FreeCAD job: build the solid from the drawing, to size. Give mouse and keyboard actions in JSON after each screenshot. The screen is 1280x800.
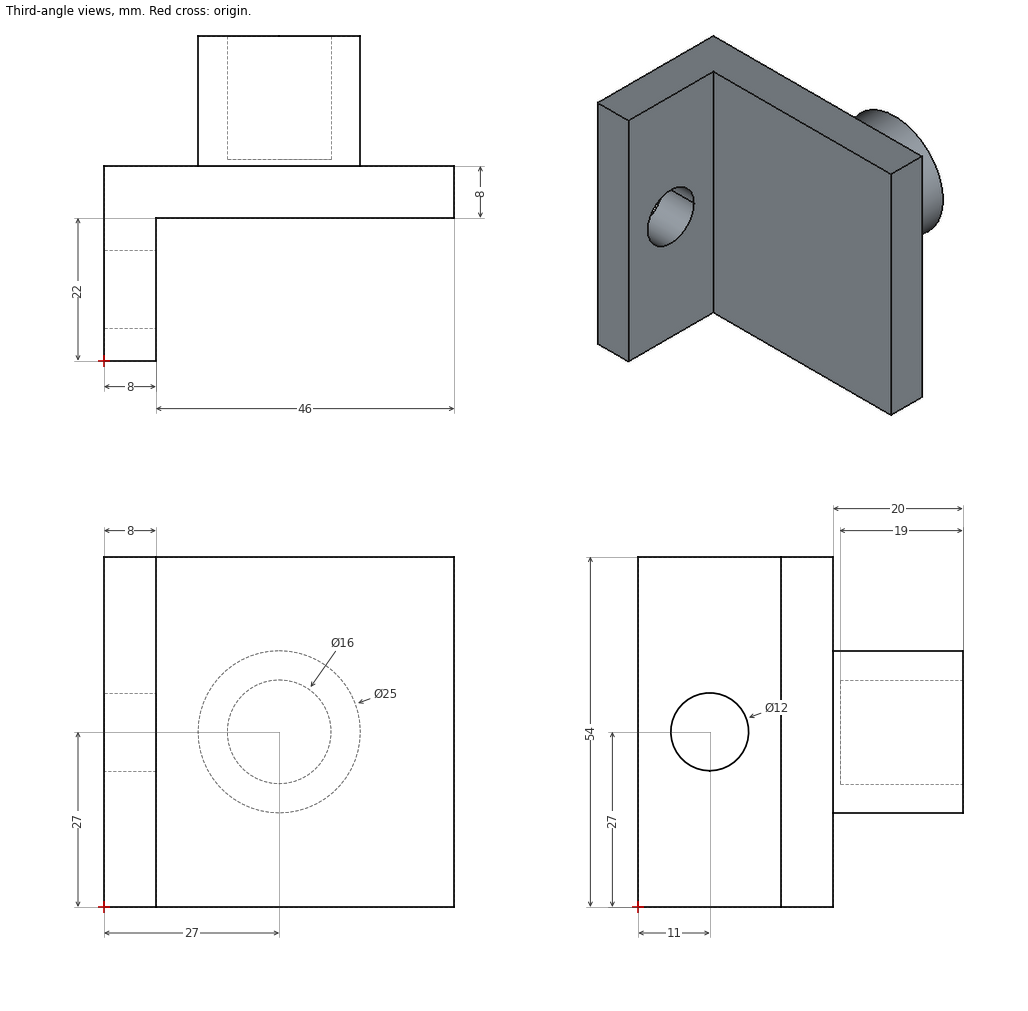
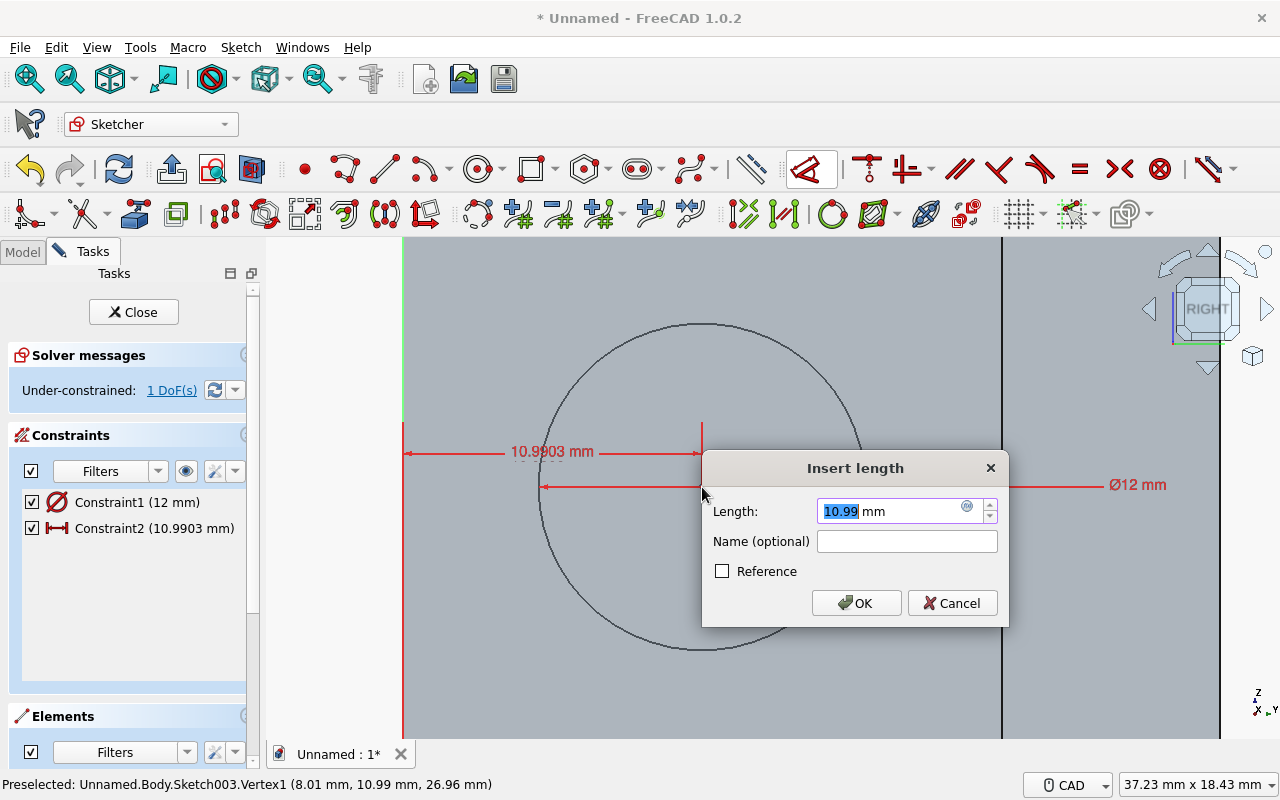
{"action": "type", "text": "11"}
{"action": "key", "text": "Return"}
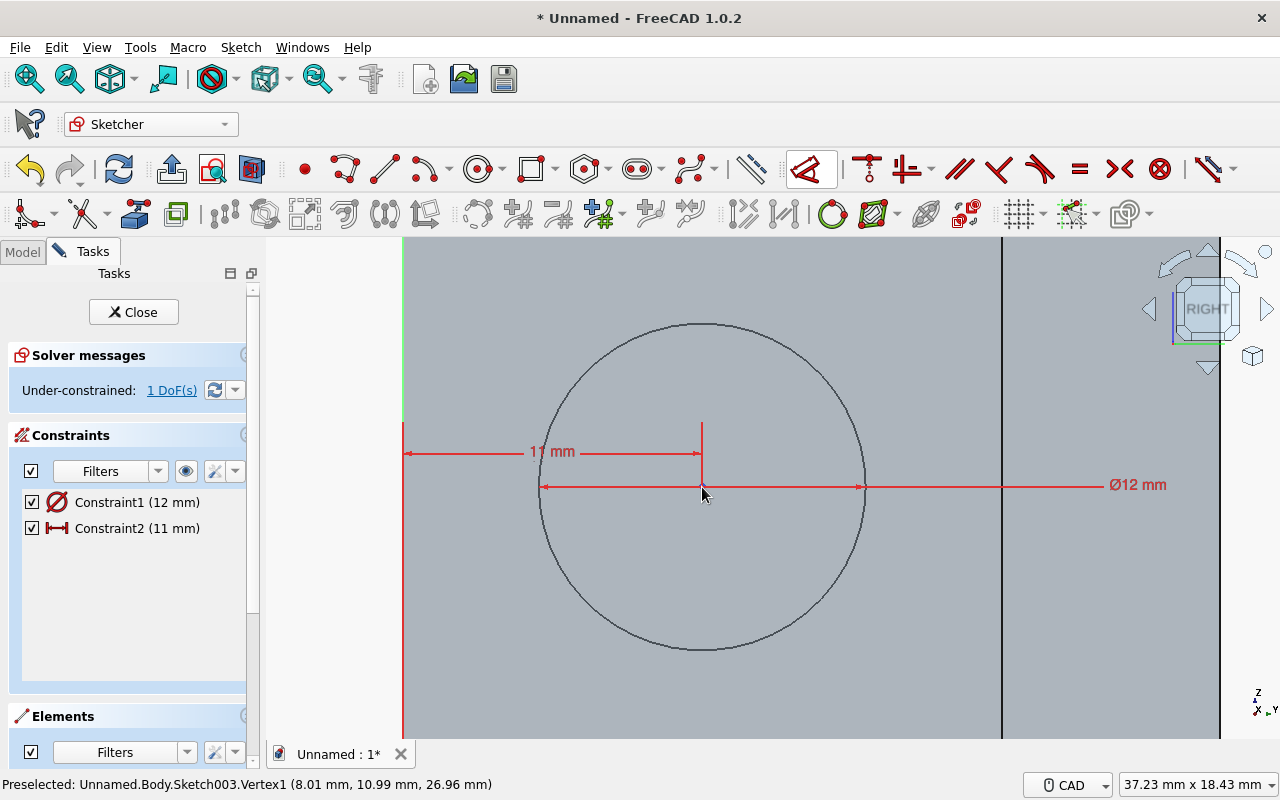
{"action": "left_click", "coordinate": [702, 487]}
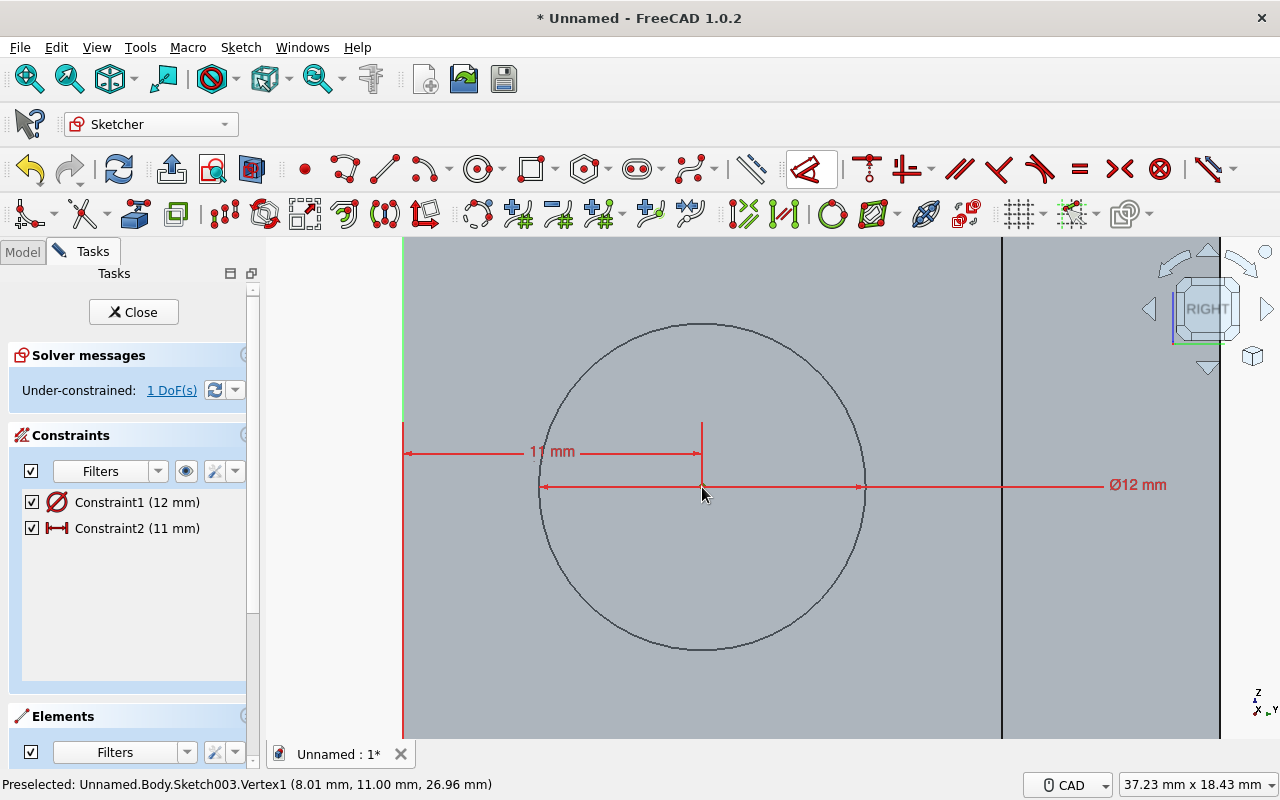
{"action": "key", "text": "i"}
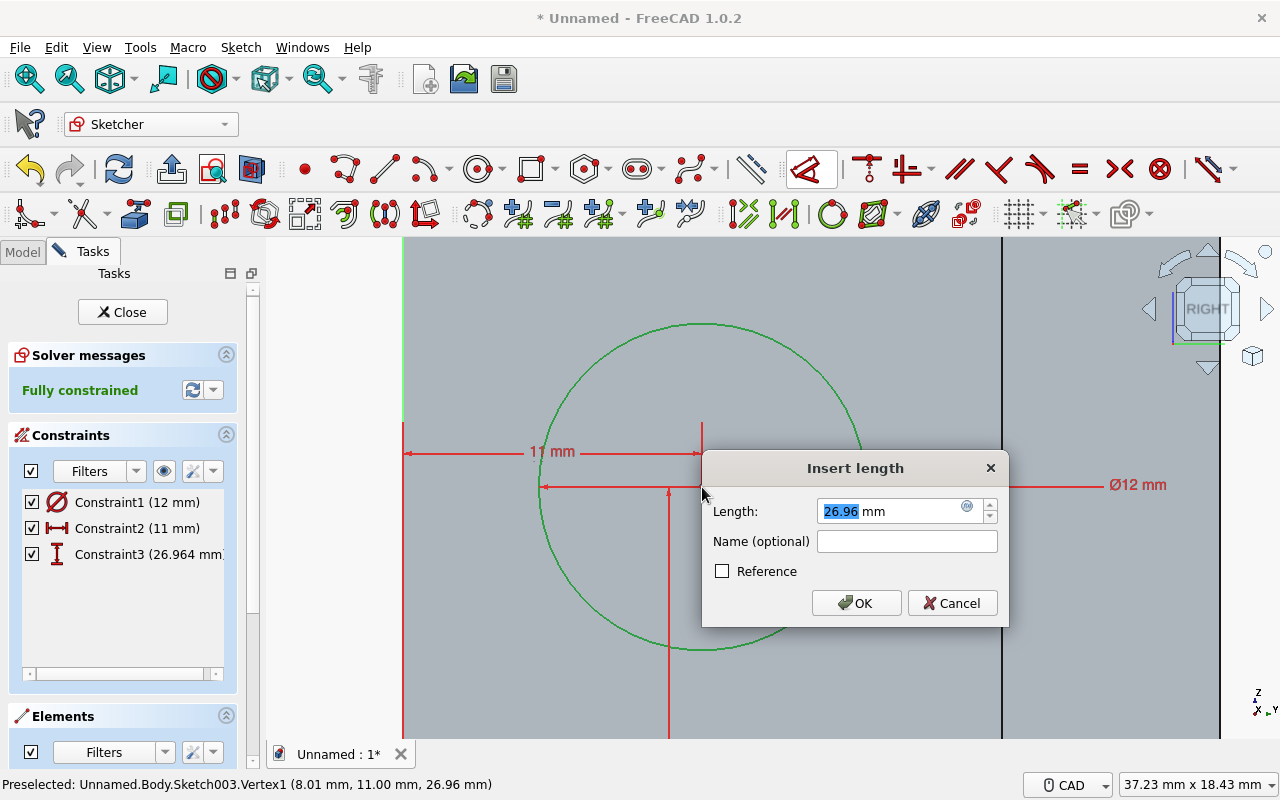
{"action": "type", "text": "27"}
{"action": "key", "text": "Return"}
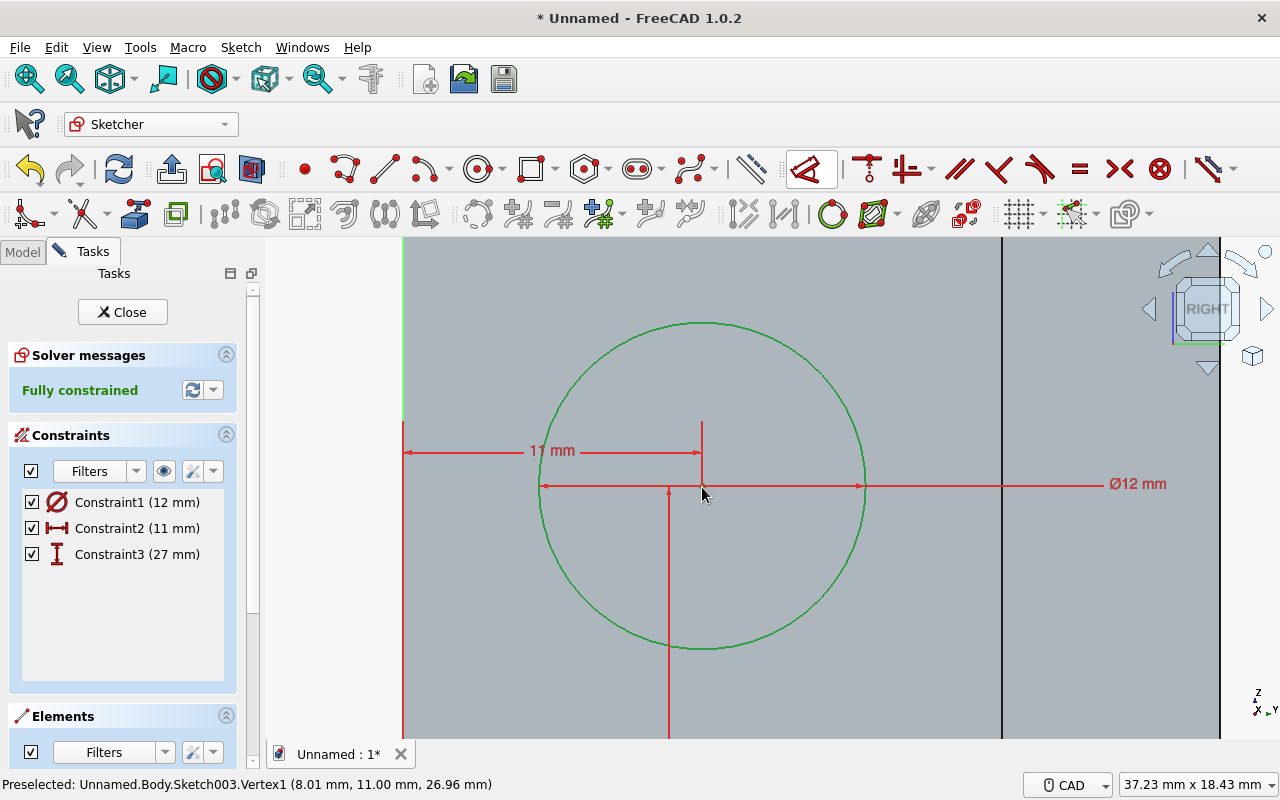
{"action": "left_click", "coordinate": [123, 312]}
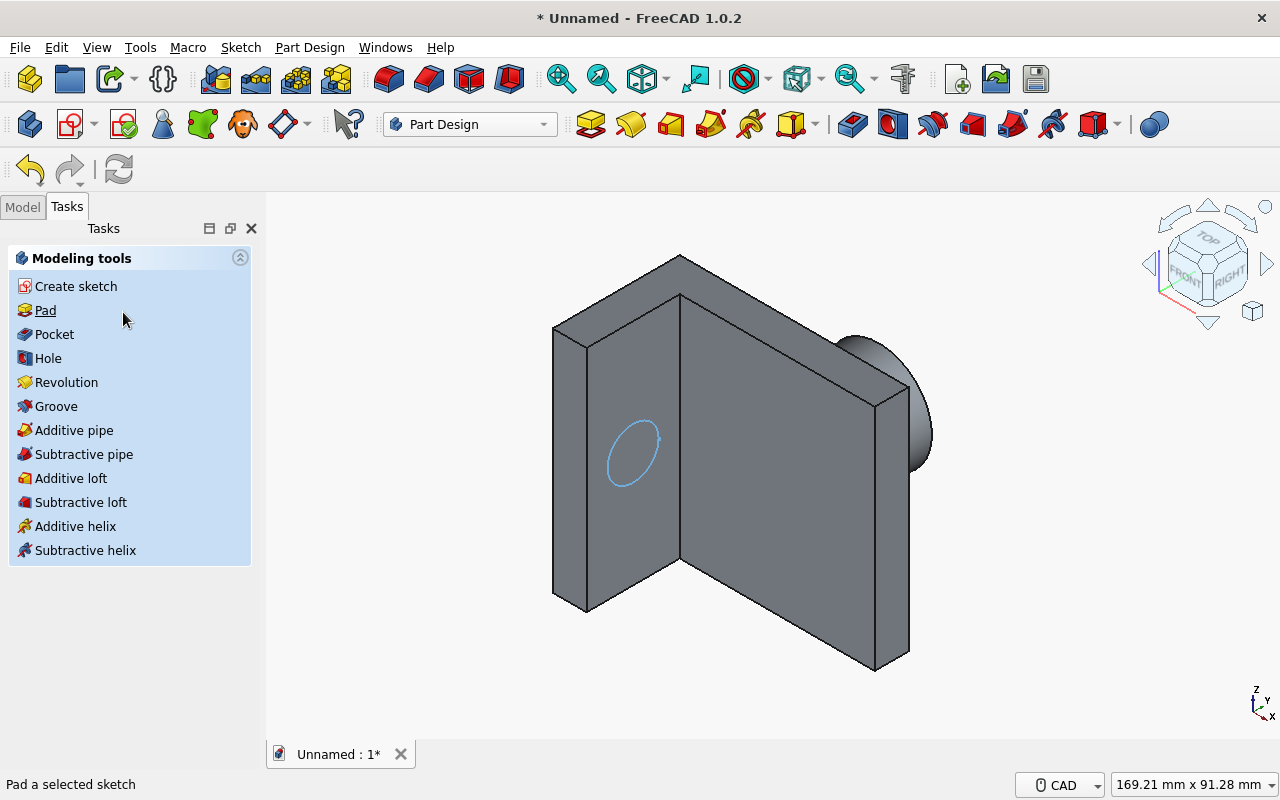
{"action": "left_click", "coordinate": [854, 124]}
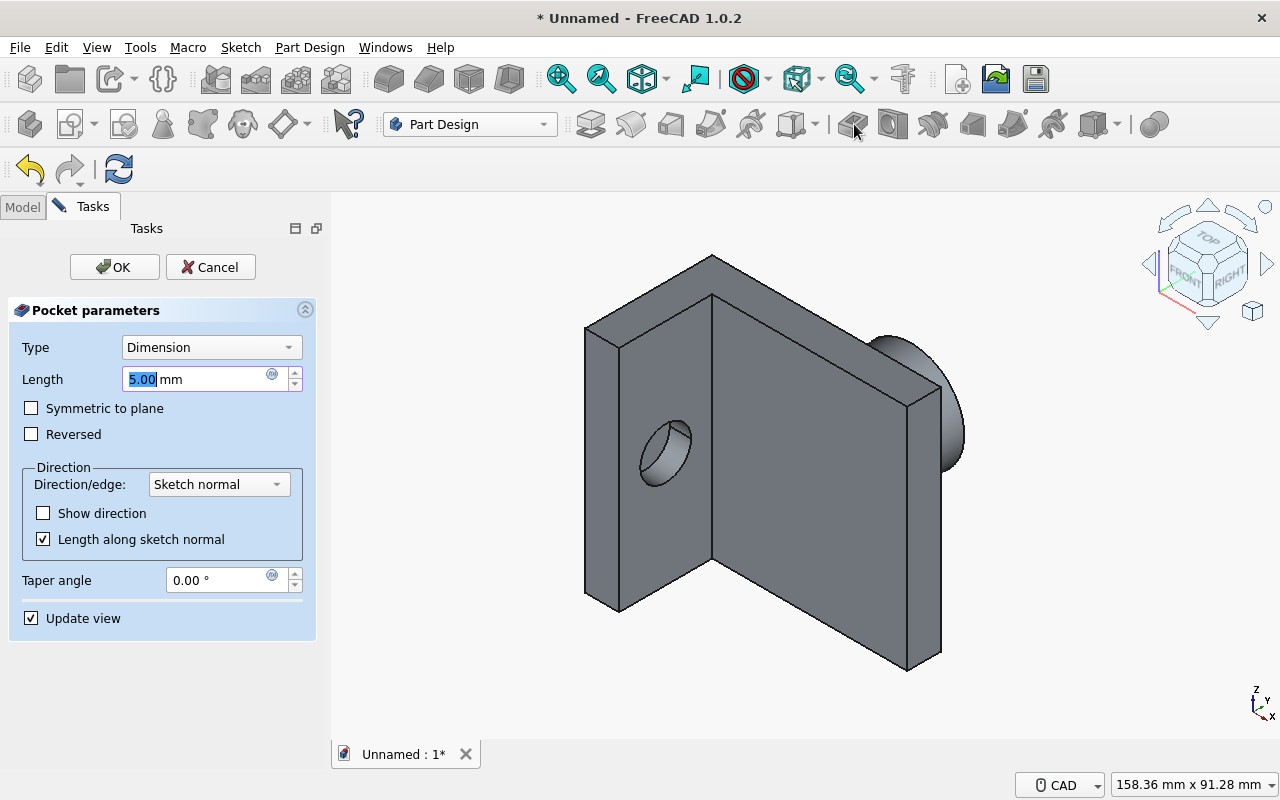
{"action": "type", "text": "8"}
{"action": "key", "text": "Tab"}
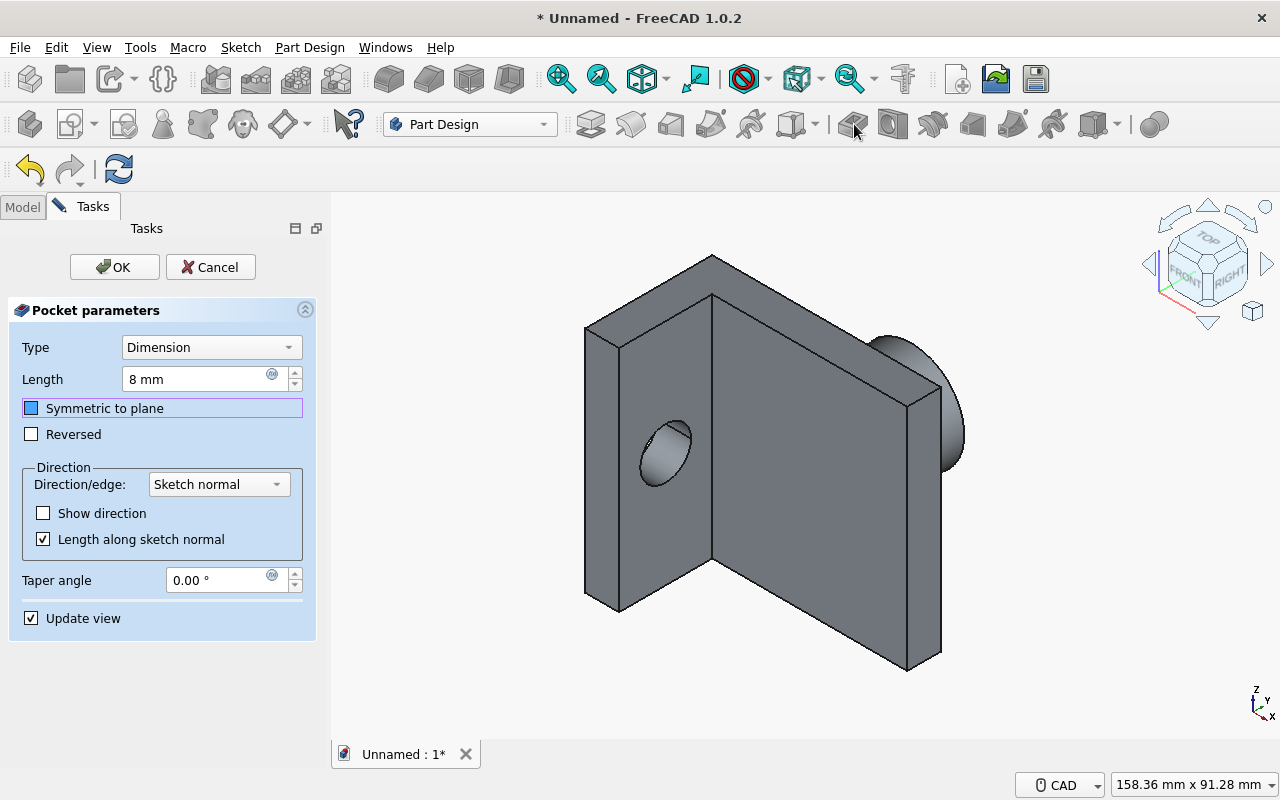
{"action": "left_click", "coordinate": [115, 267]}